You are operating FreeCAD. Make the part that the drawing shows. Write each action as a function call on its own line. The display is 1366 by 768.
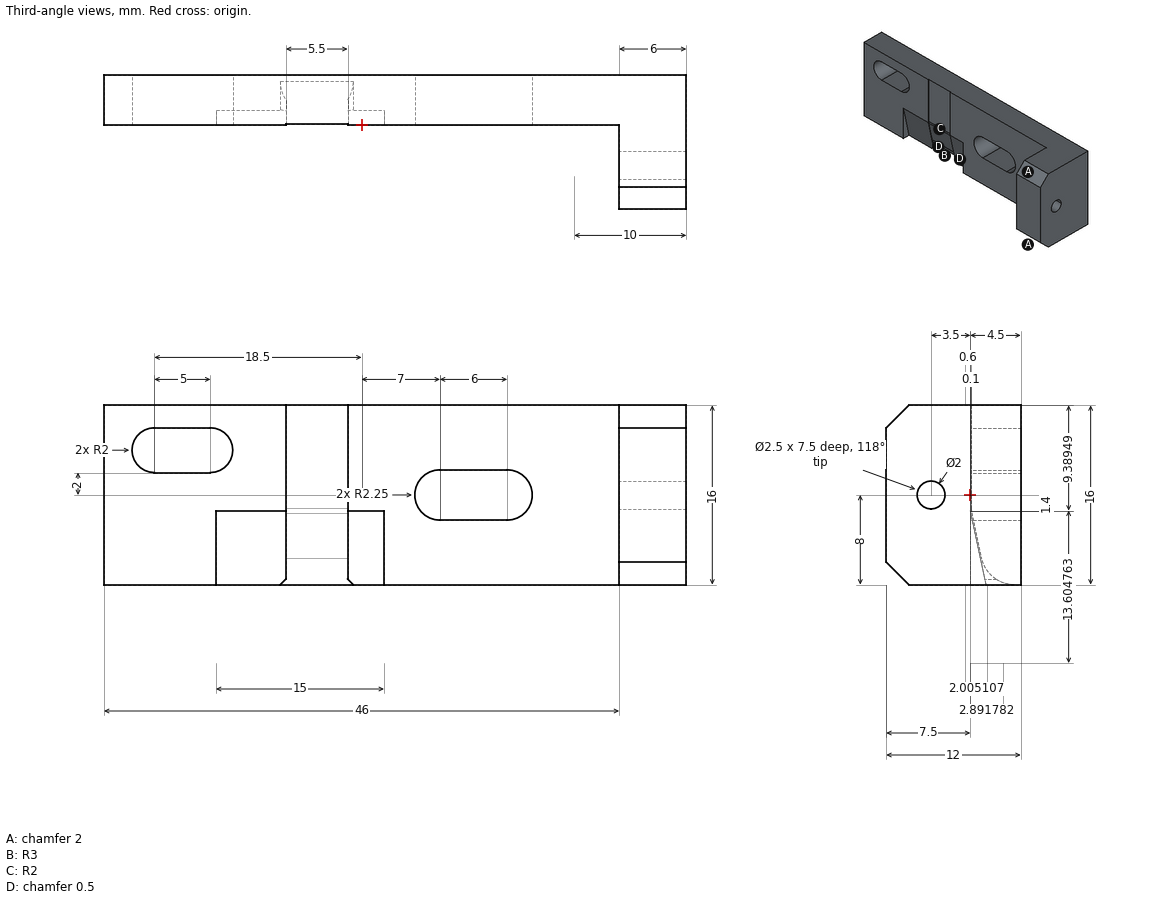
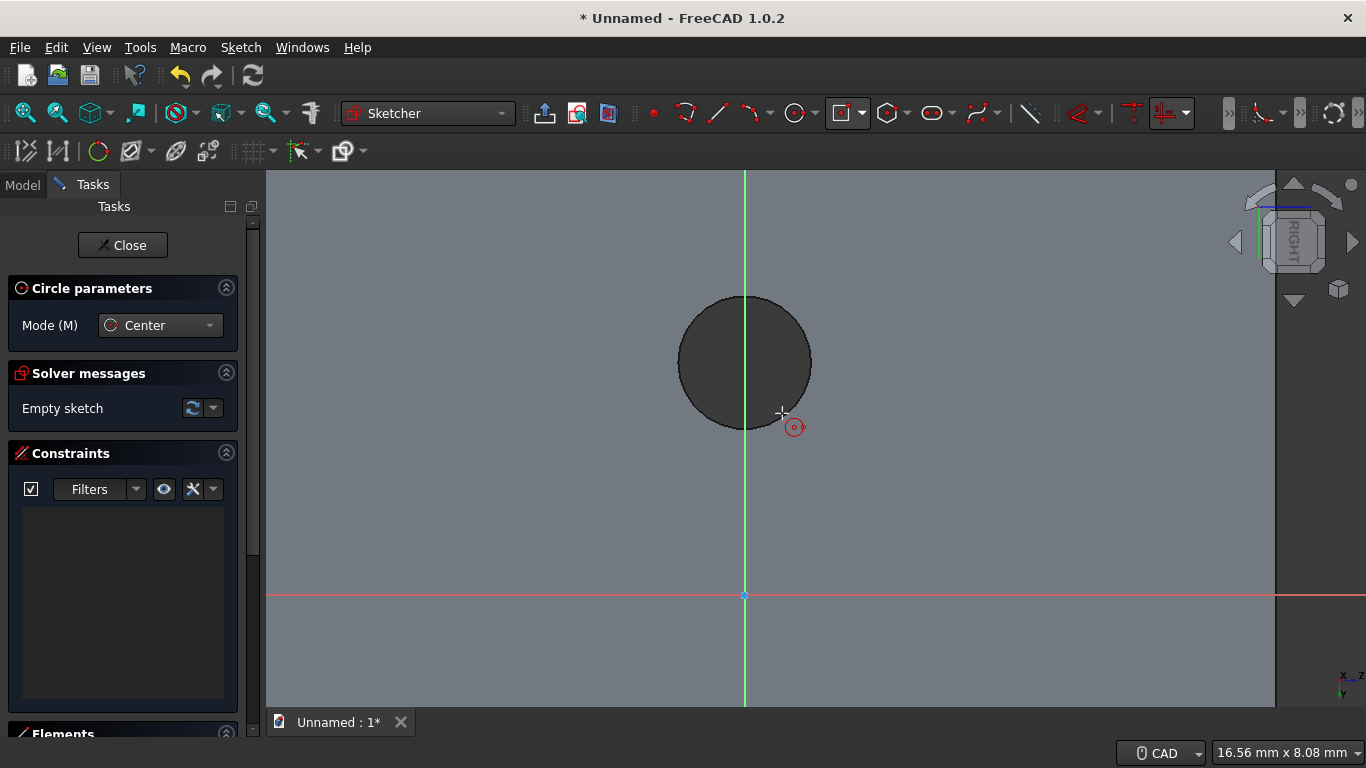
click(745, 363)
click(803, 304)
key(Escape)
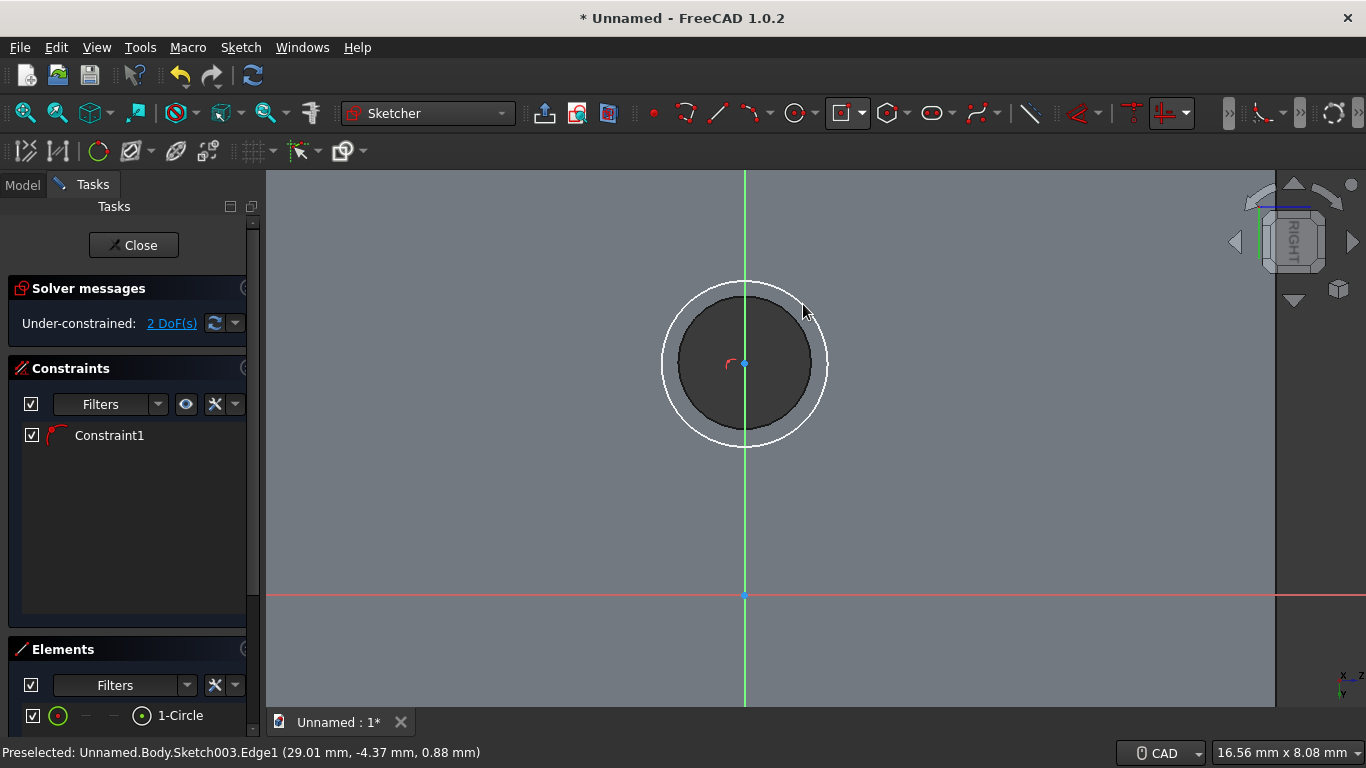
key(d)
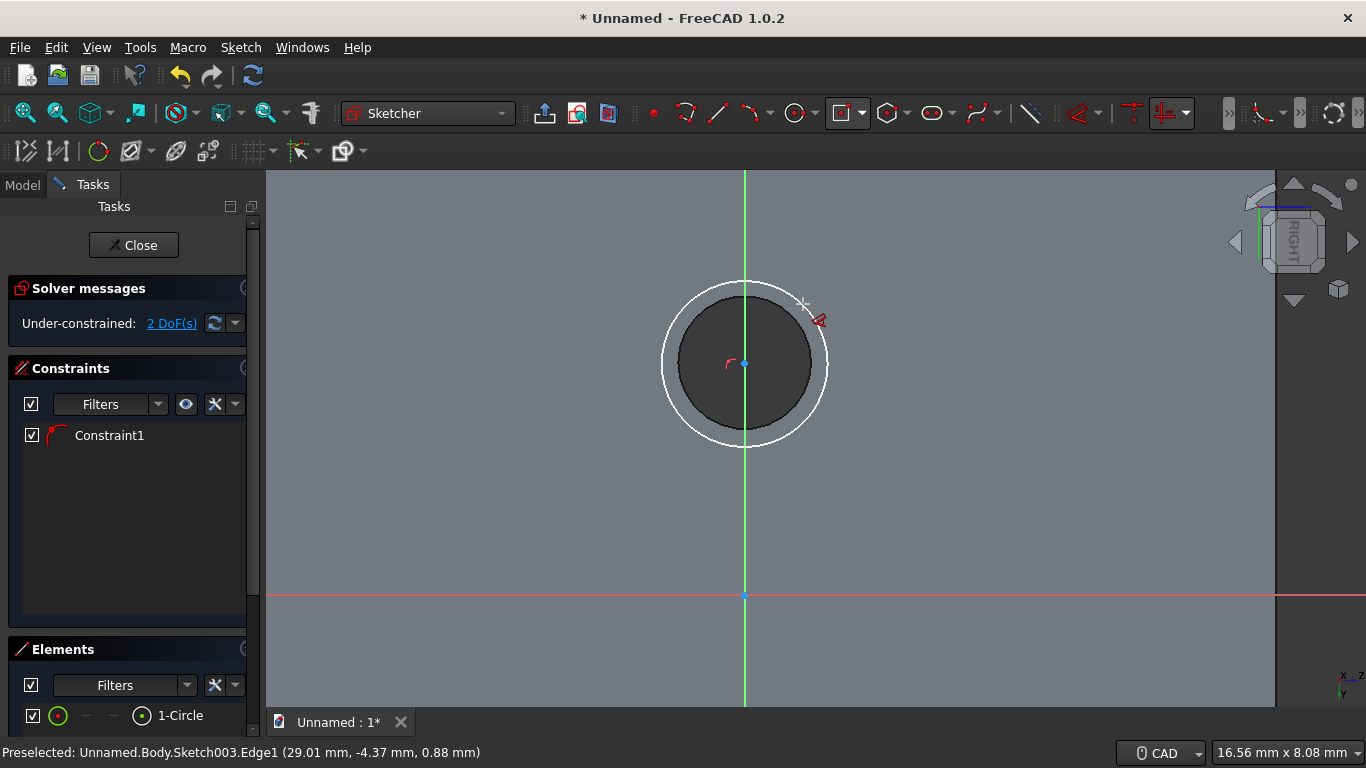
click(803, 305)
click(825, 282)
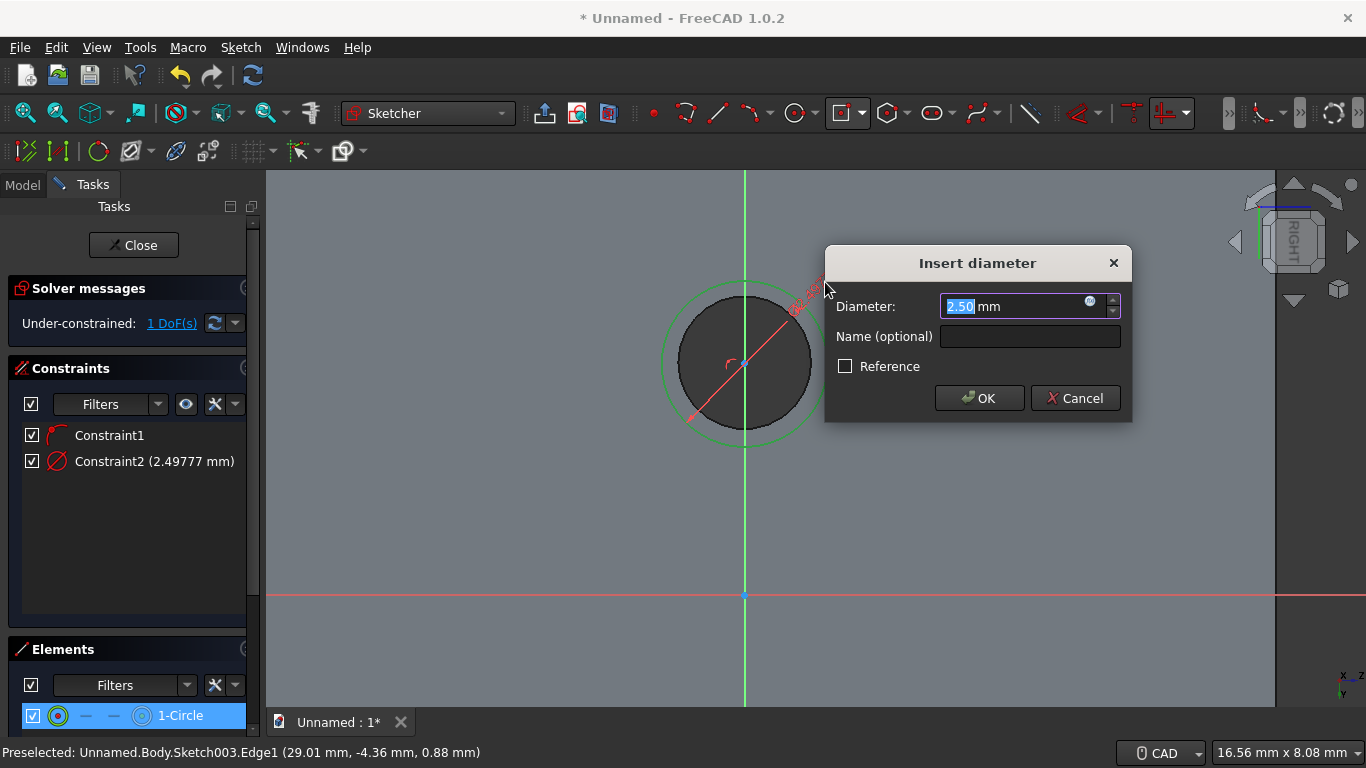
text(2.5)
key(Return)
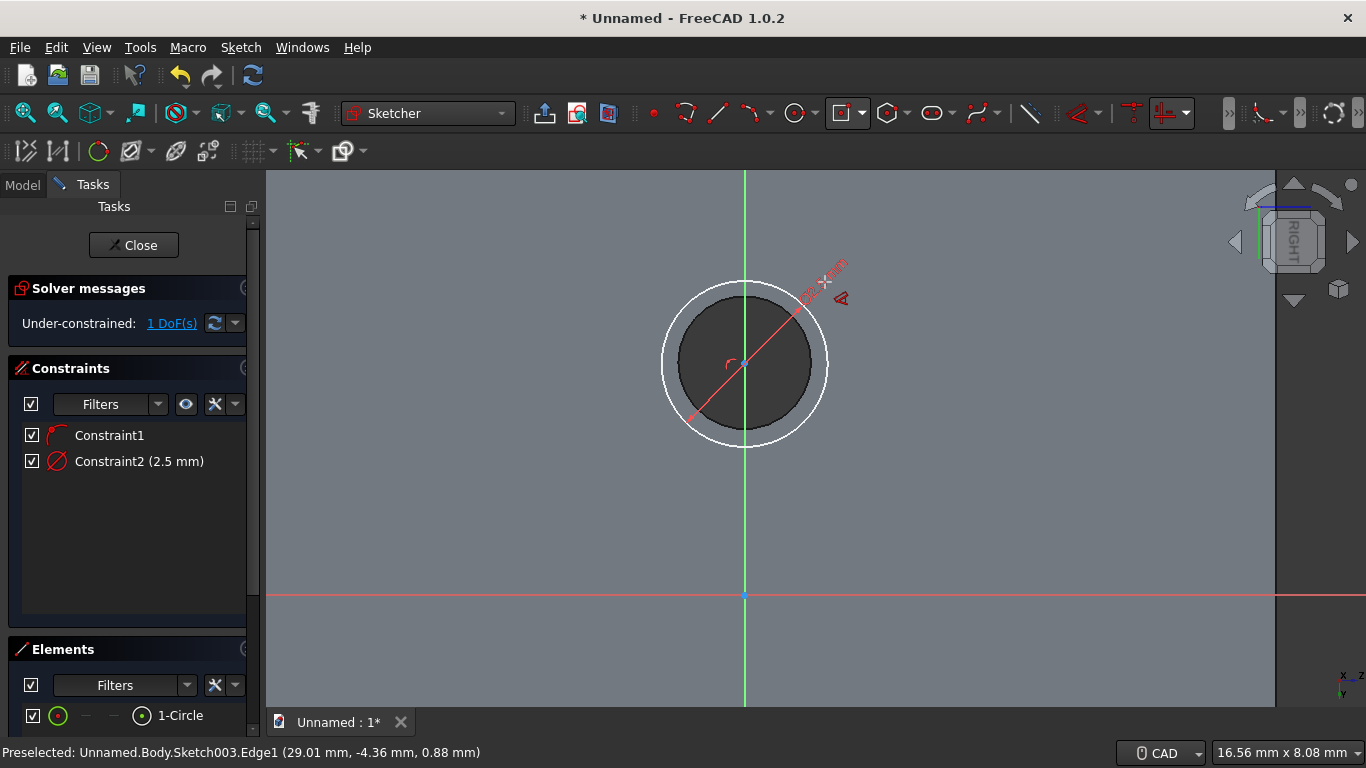
click(747, 366)
click(779, 480)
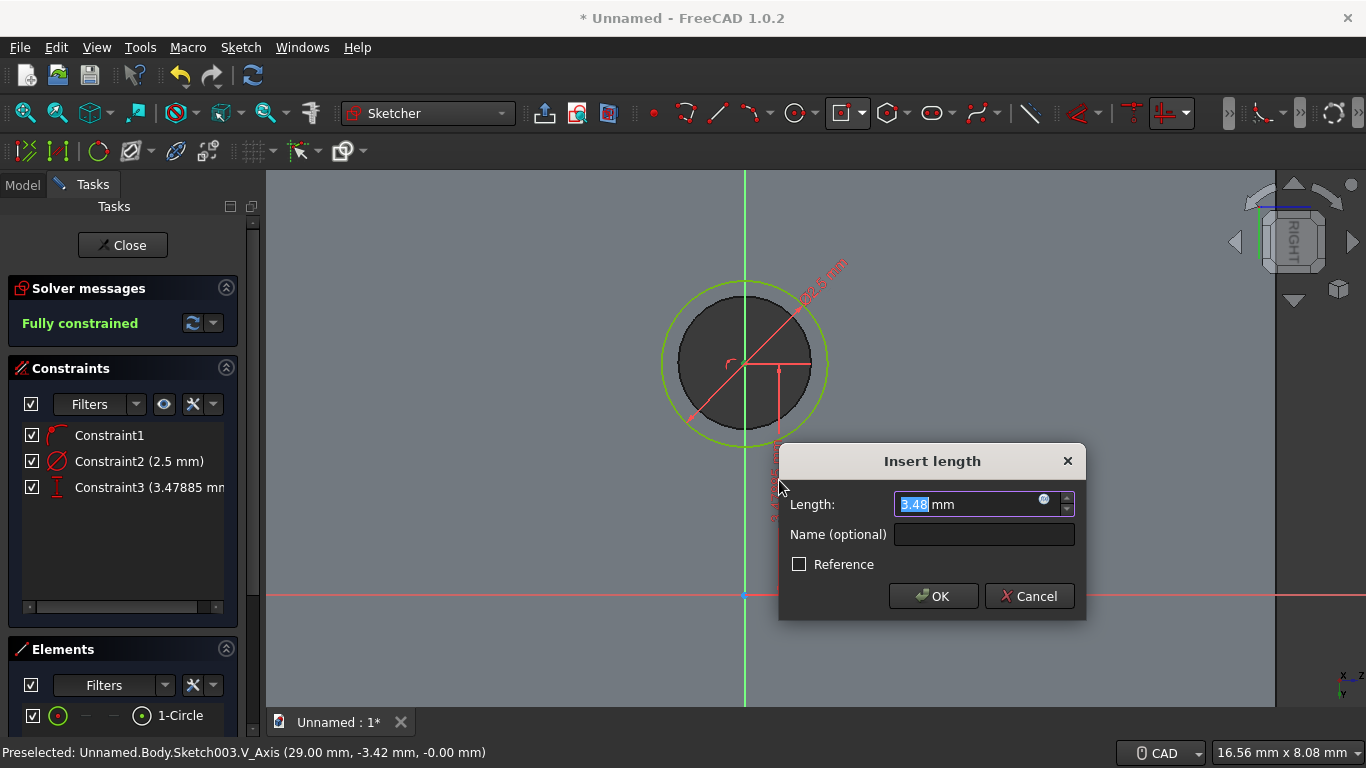
text(3.5)
key(Return)
key(Escape)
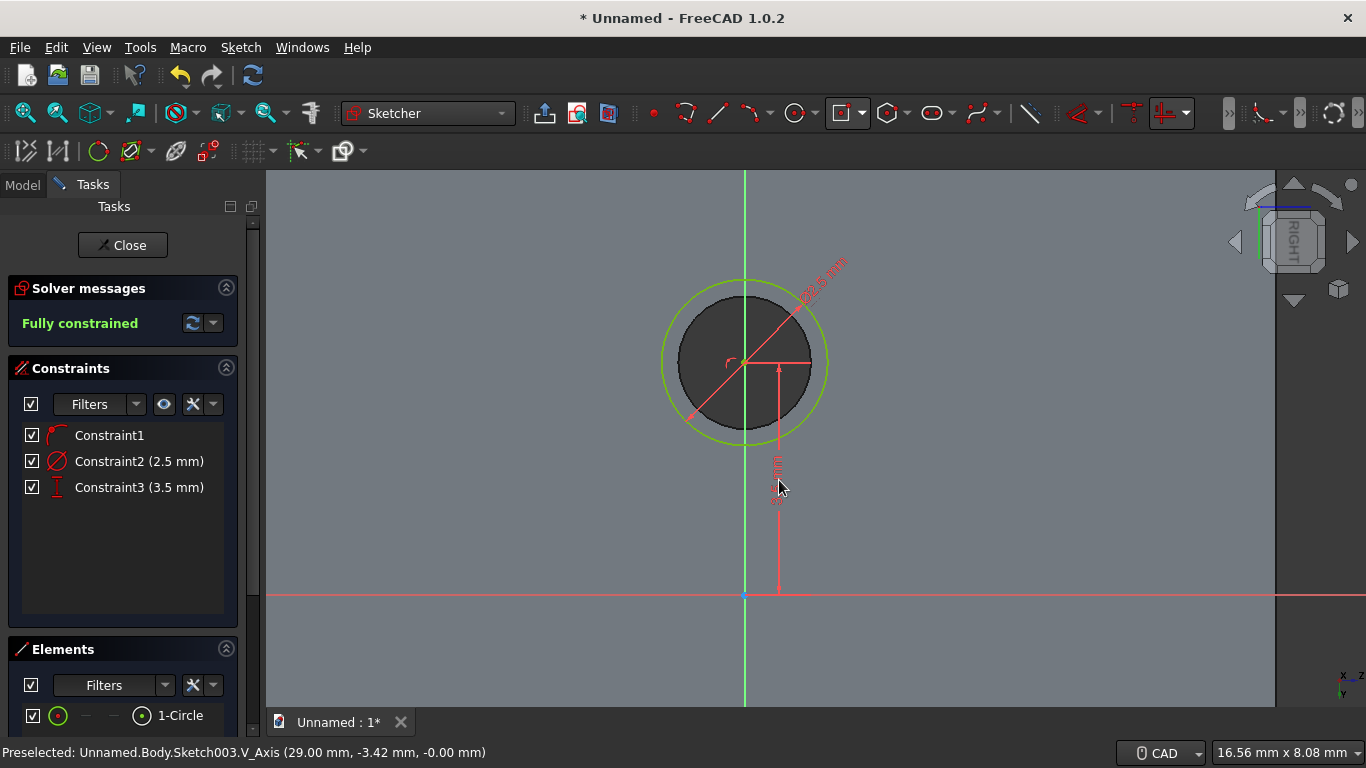
click(123, 245)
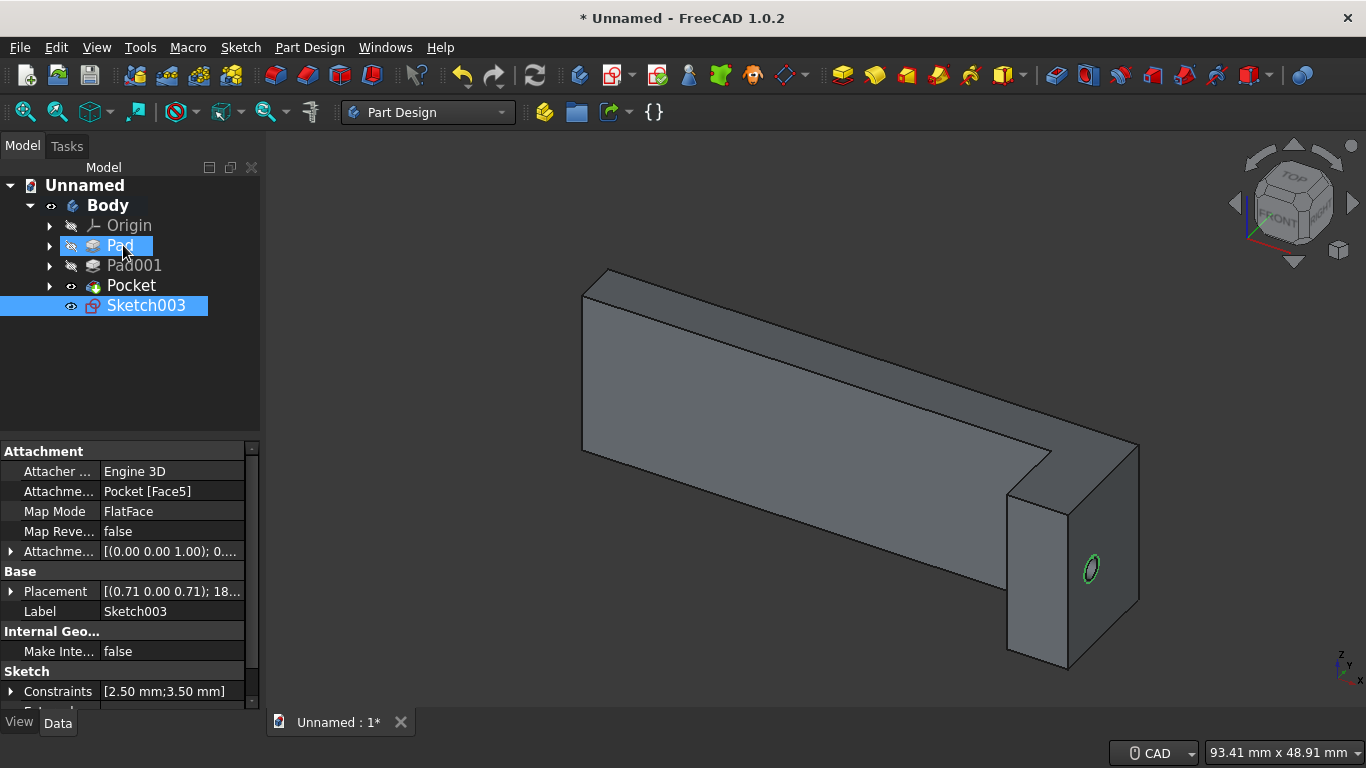
click(1090, 76)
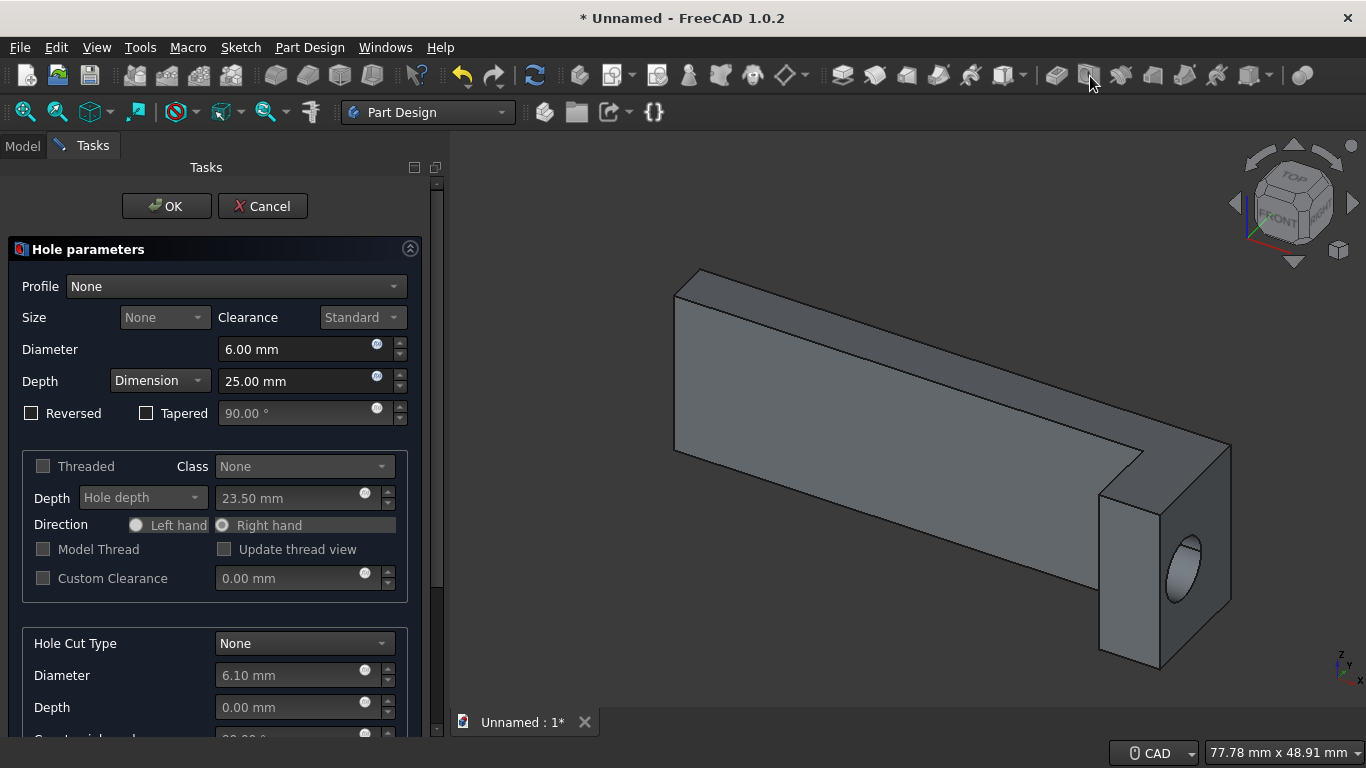
triple_click(305, 349)